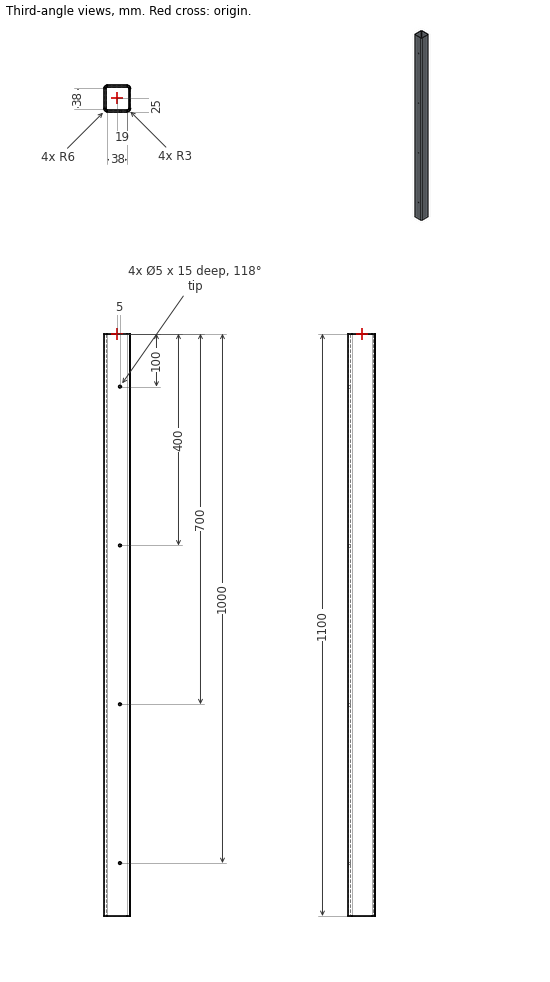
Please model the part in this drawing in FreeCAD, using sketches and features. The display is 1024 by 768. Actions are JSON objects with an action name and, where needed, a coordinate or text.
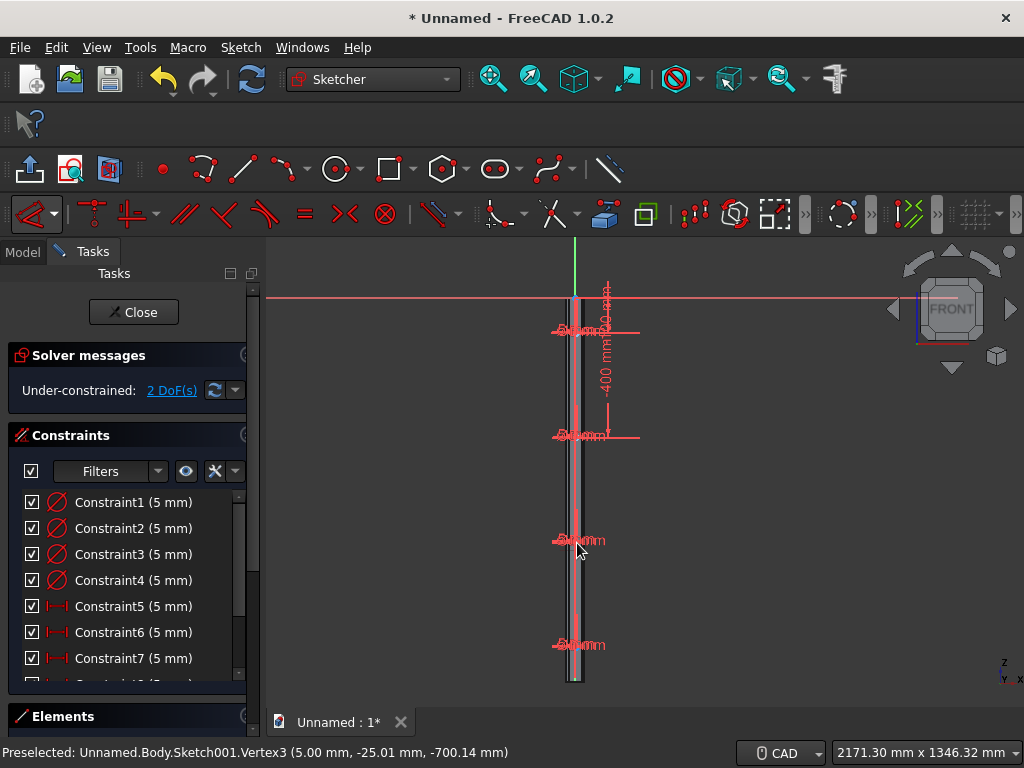
{"action": "key", "text": "i"}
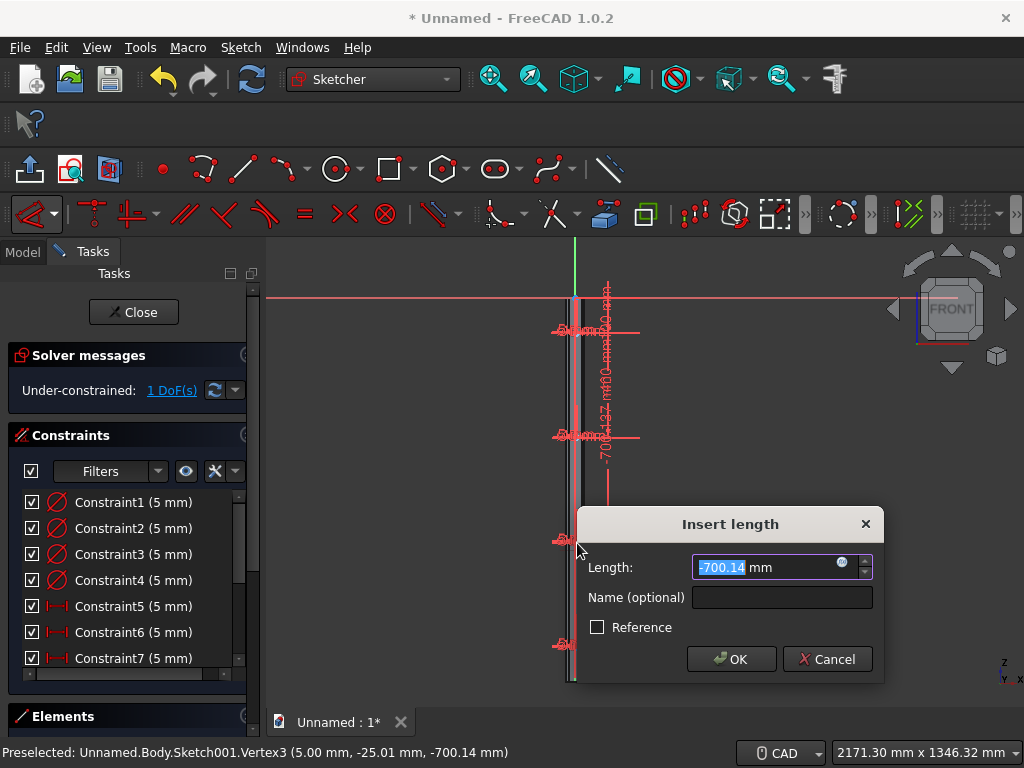
{"action": "type", "text": "-700"}
{"action": "key", "text": "Return"}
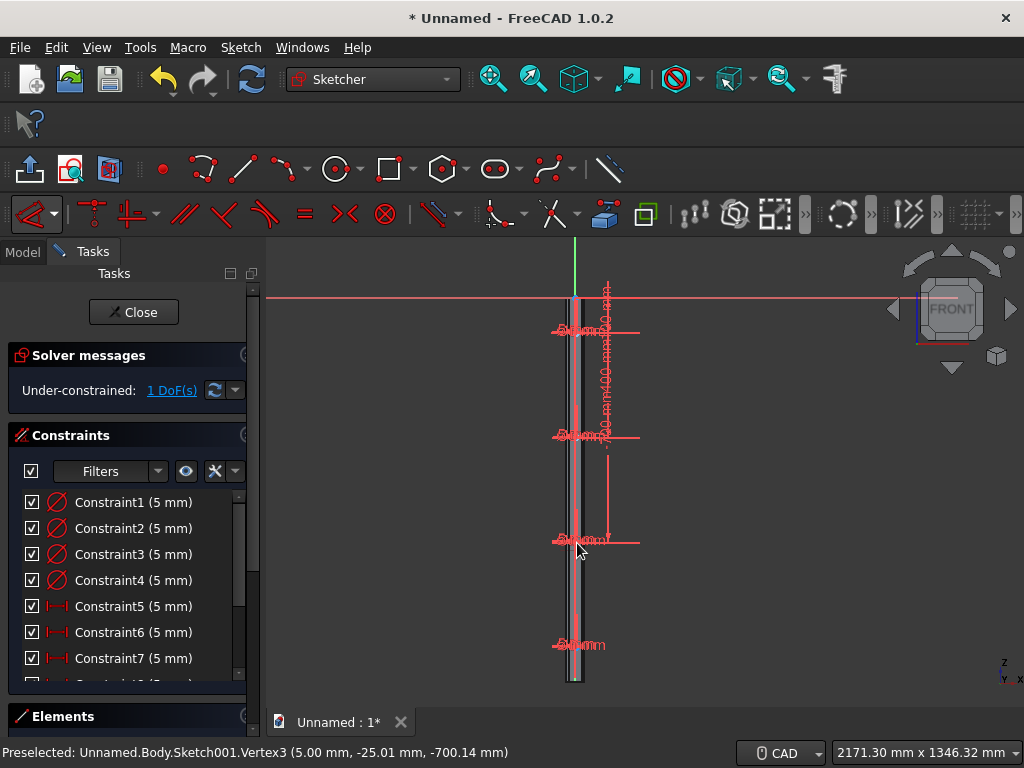
{"action": "left_click", "coordinate": [577, 647]}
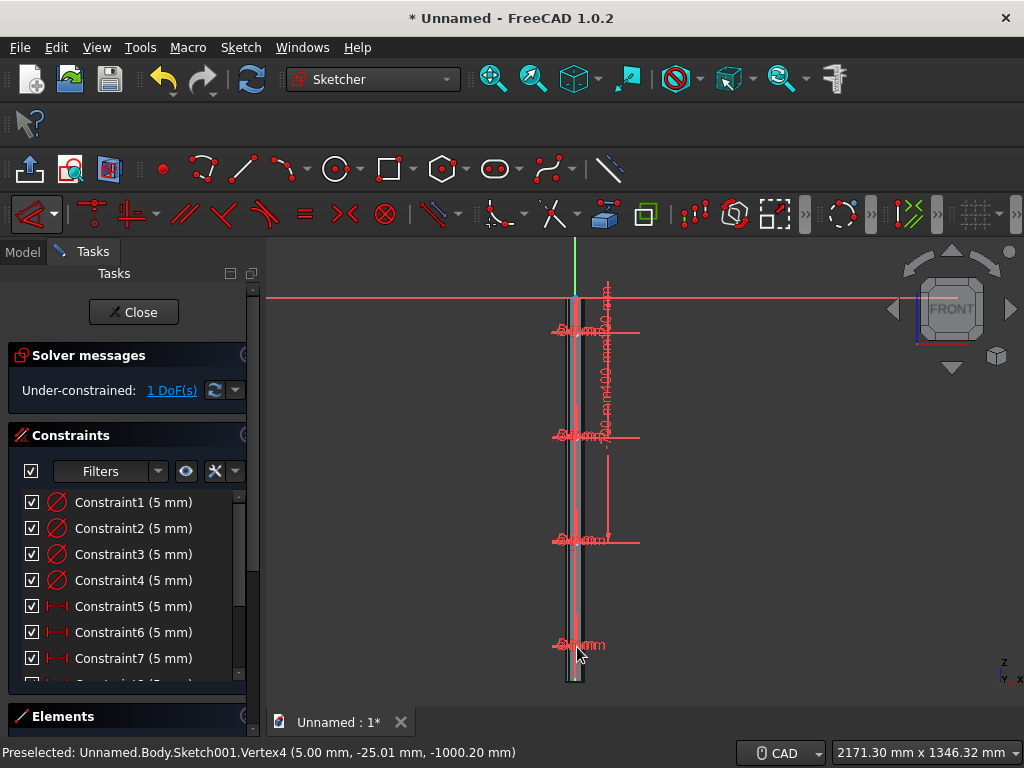
{"action": "left_click", "coordinate": [56, 214]}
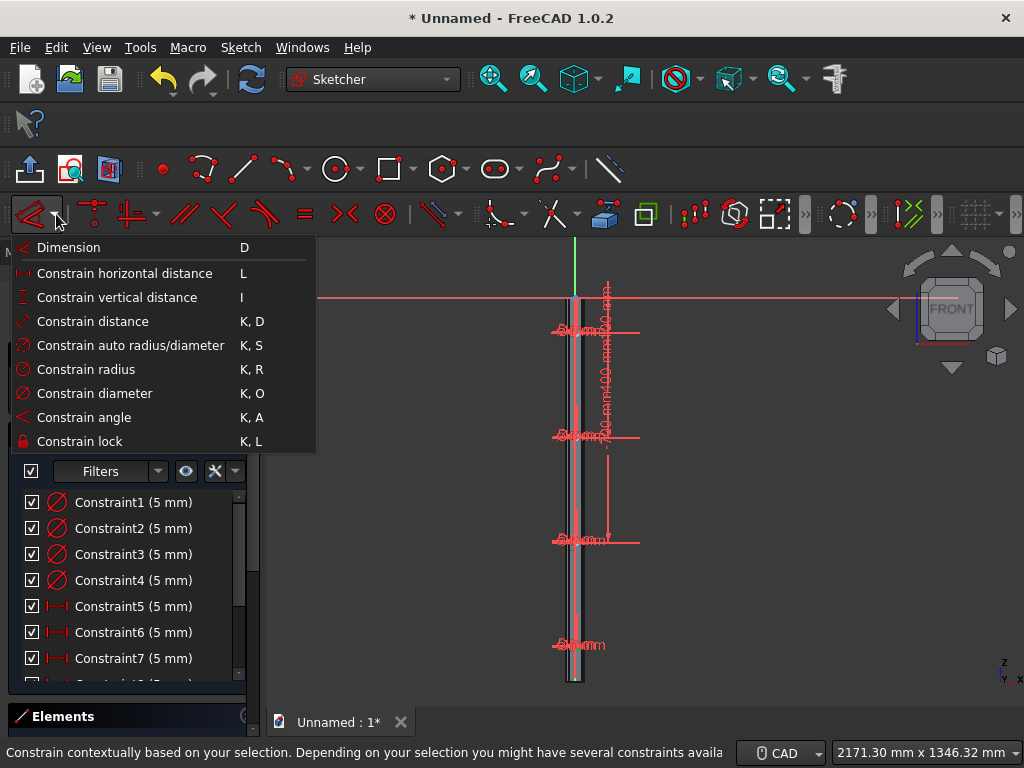
{"action": "left_click", "coordinate": [164, 297]}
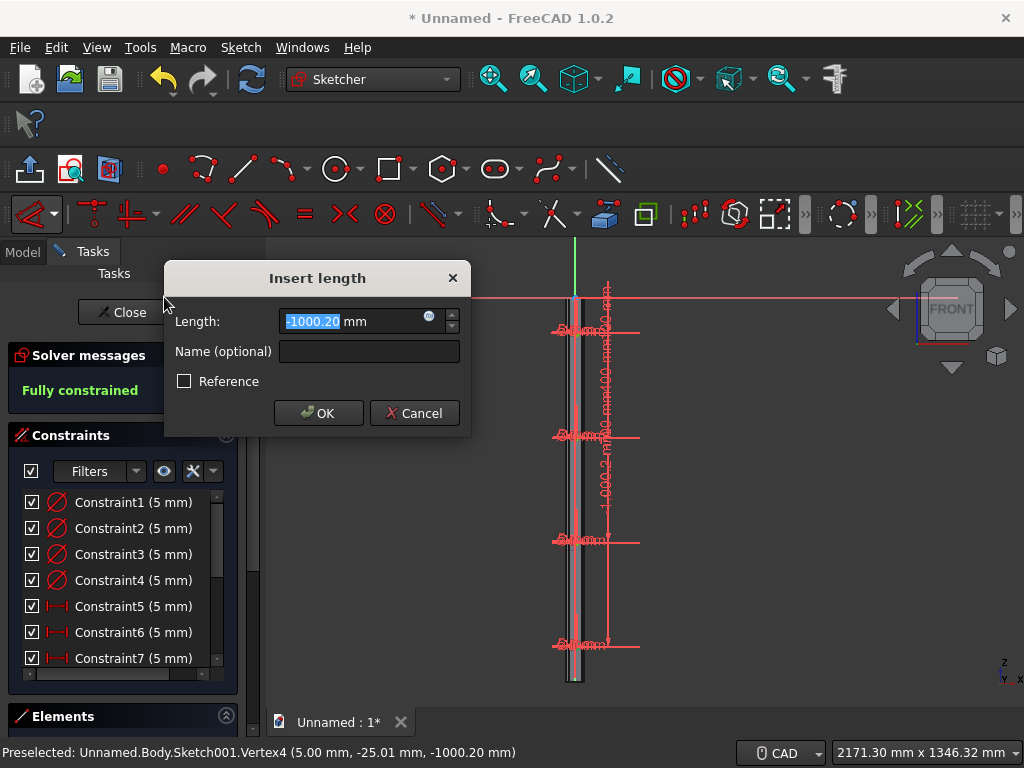
{"action": "type", "text": "-1000"}
{"action": "key", "text": "Return"}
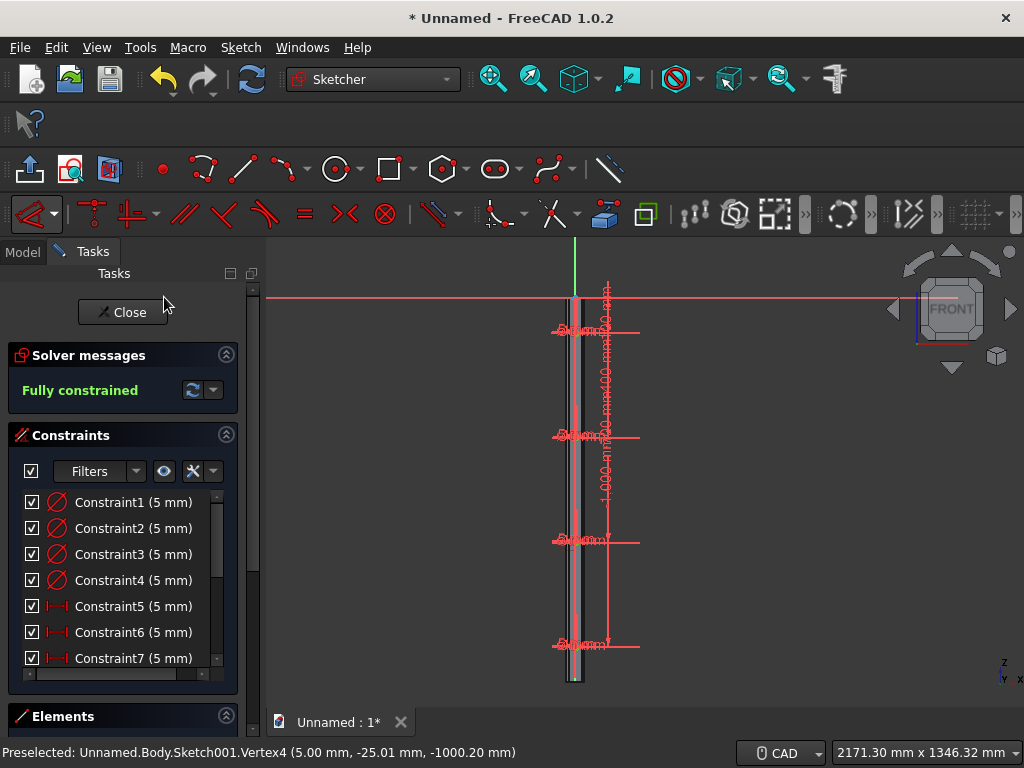
{"action": "left_click", "coordinate": [123, 312]}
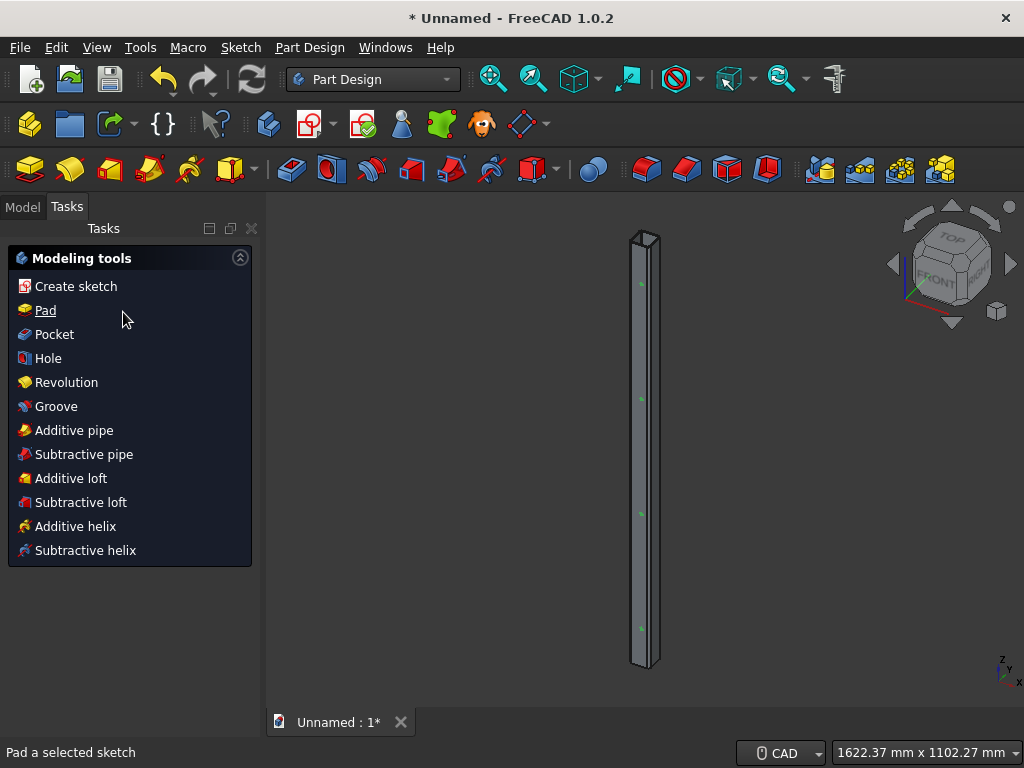
{"action": "left_click", "coordinate": [332, 170]}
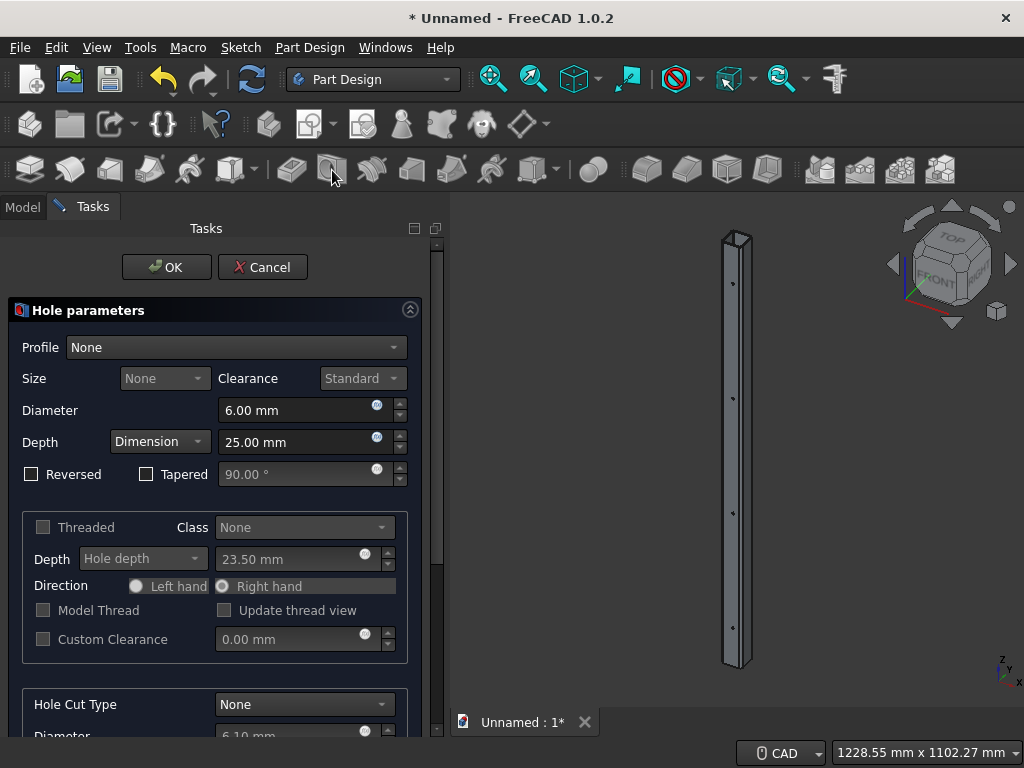
{"action": "triple_click", "coordinate": [305, 410]}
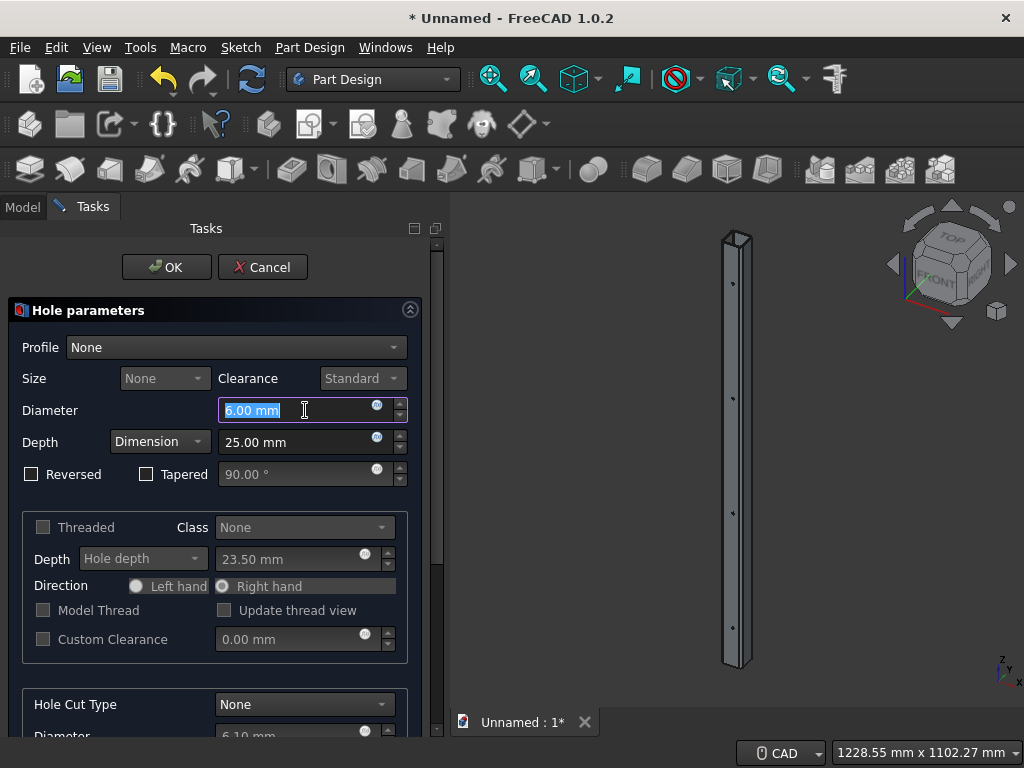
{"action": "type", "text": "5"}
{"action": "key", "text": "Tab"}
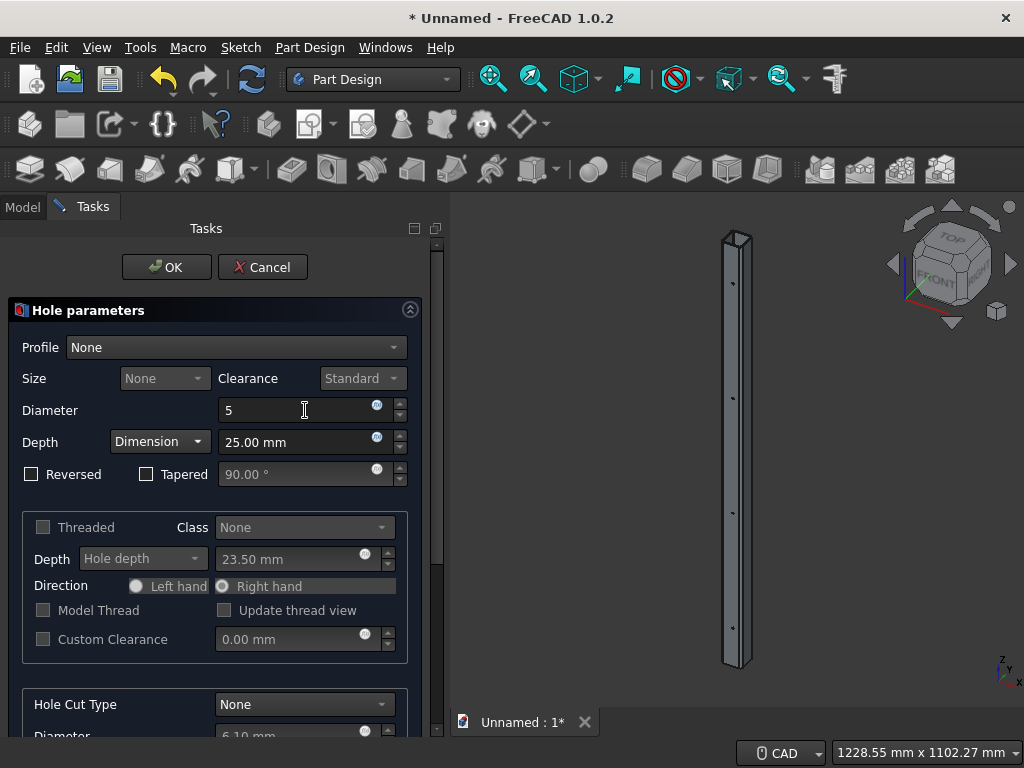
{"action": "triple_click", "coordinate": [305, 442]}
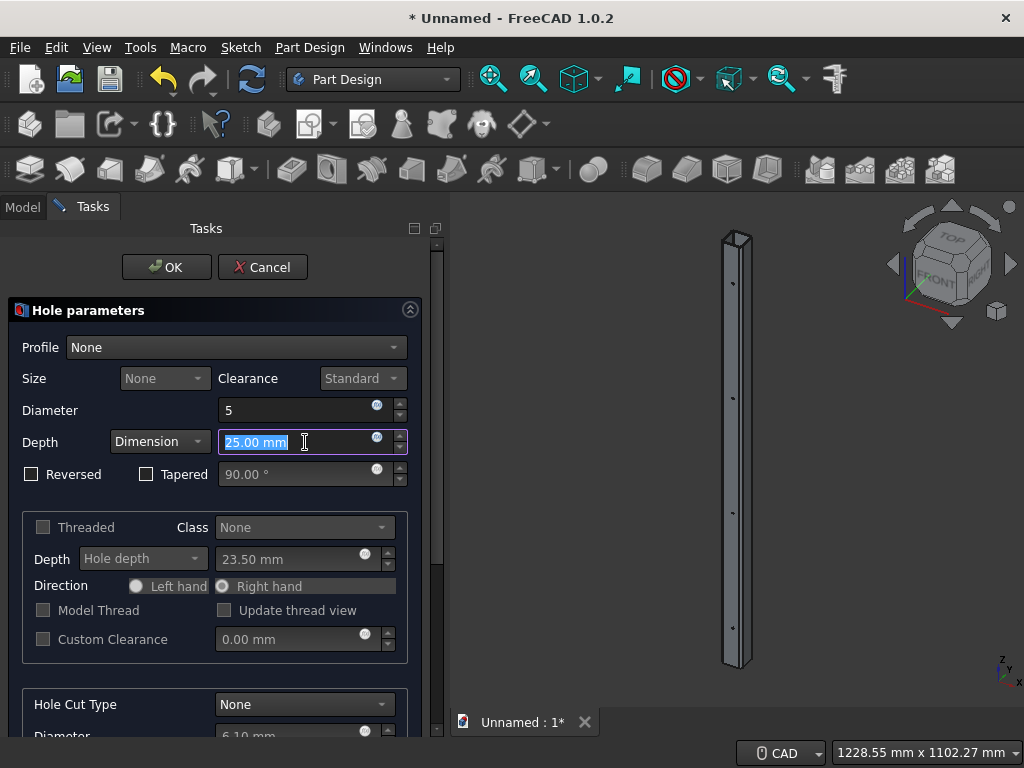
{"action": "type", "text": "15"}
{"action": "key", "text": "Tab"}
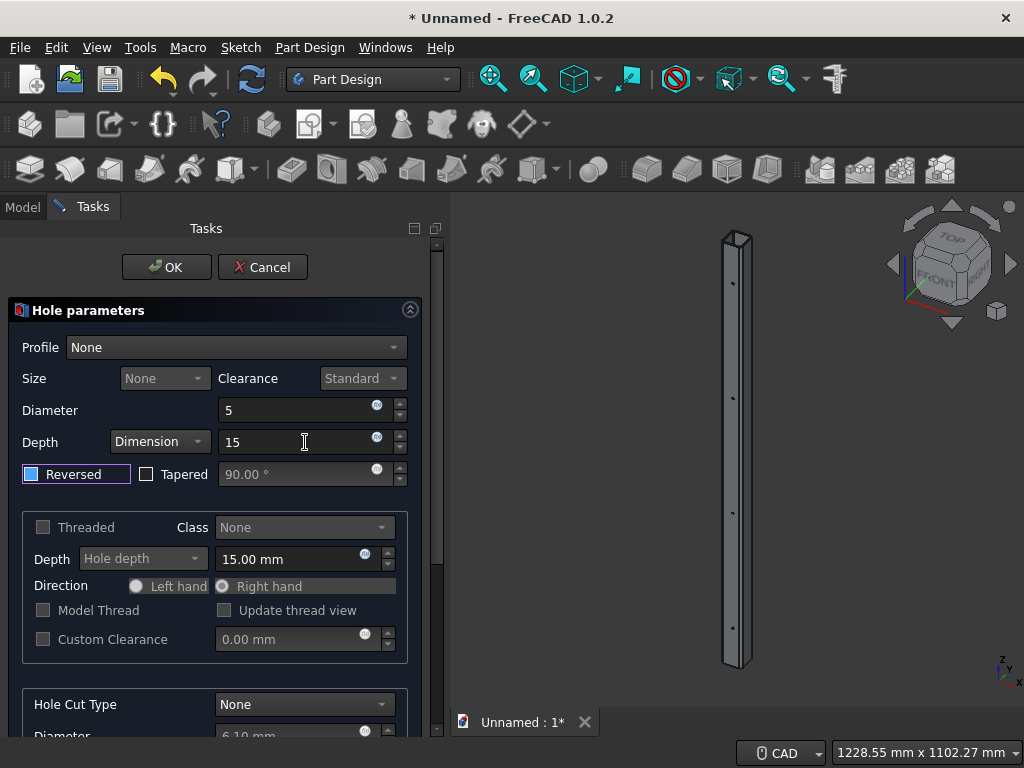
{"action": "left_click", "coordinate": [167, 267]}